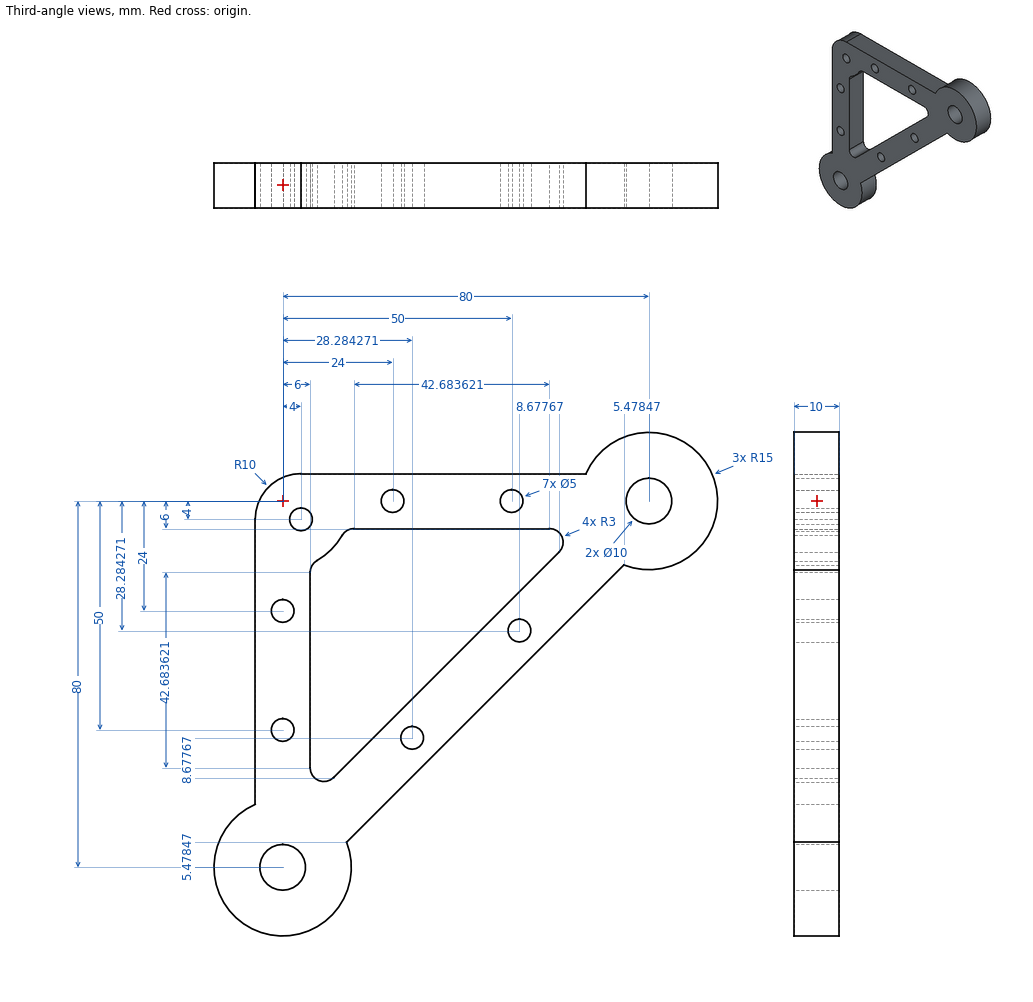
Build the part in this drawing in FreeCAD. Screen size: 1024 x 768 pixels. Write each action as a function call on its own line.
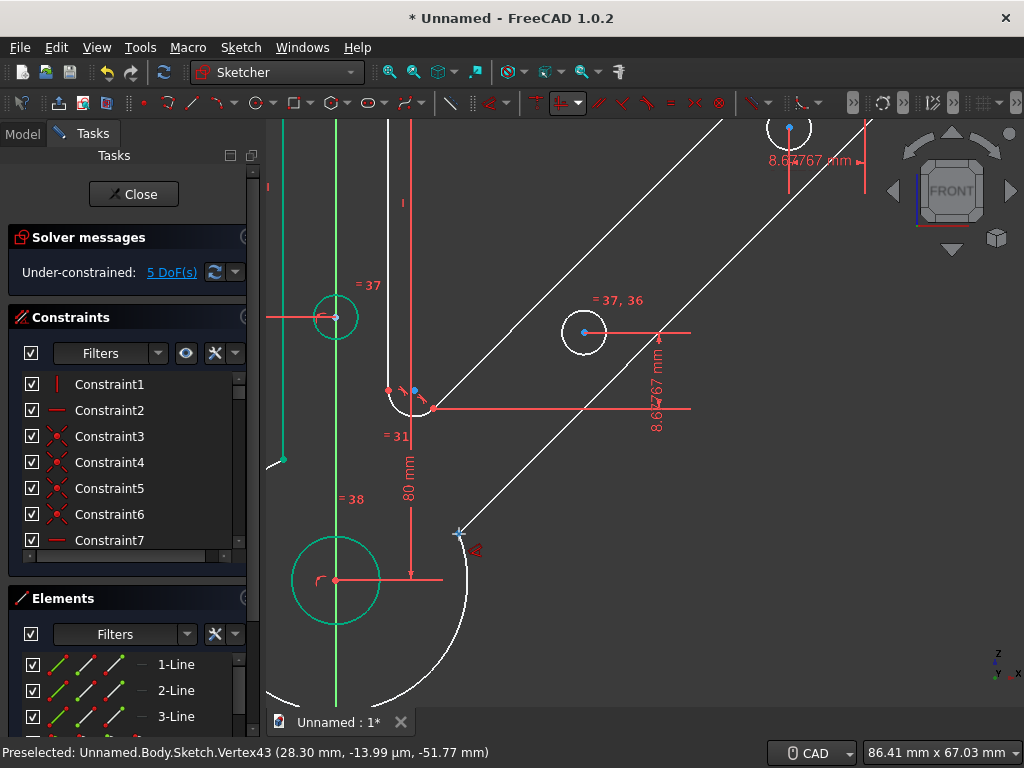
click(459, 534)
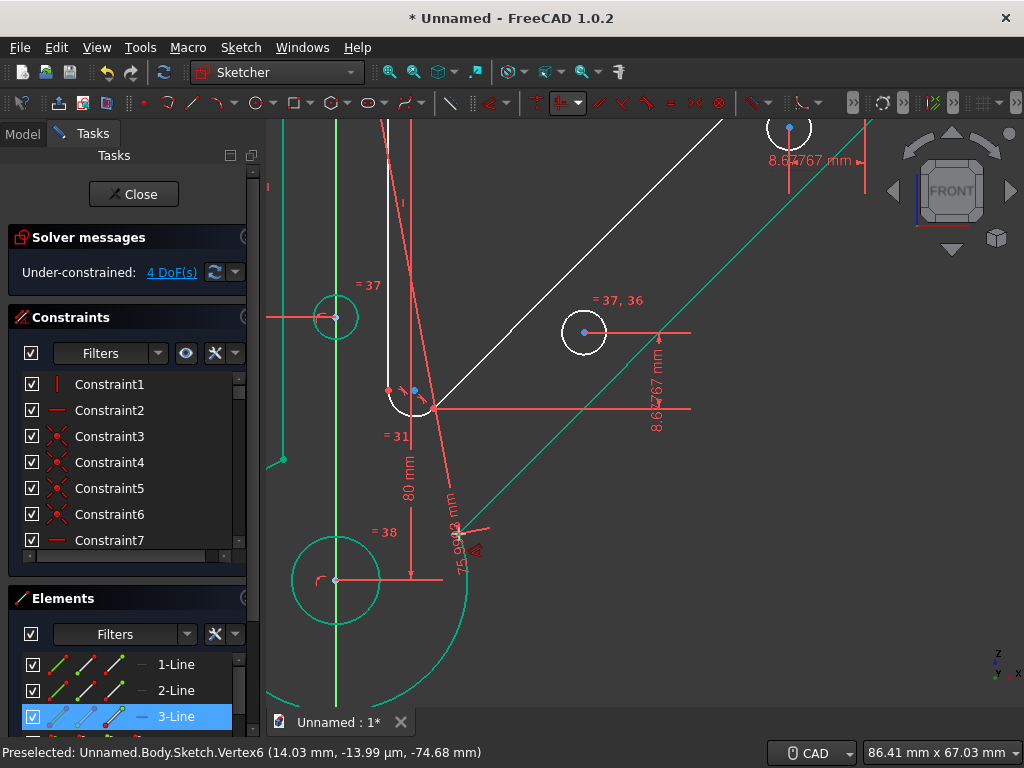
click(336, 580)
click(493, 557)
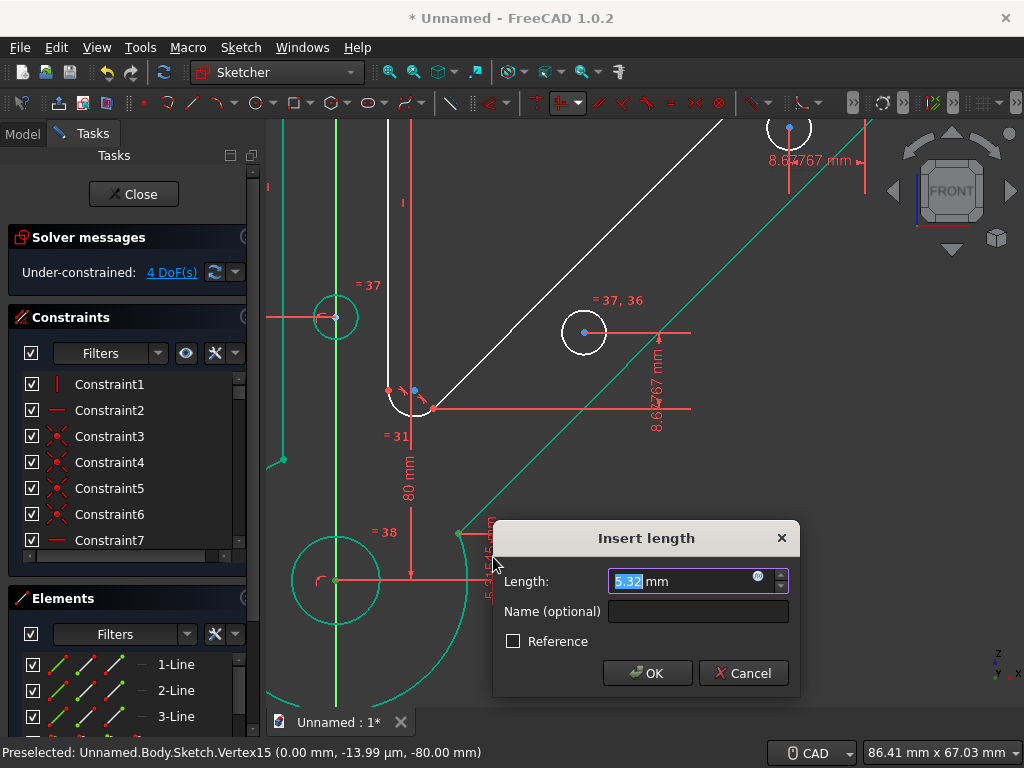
text(5.47847)
key(Return)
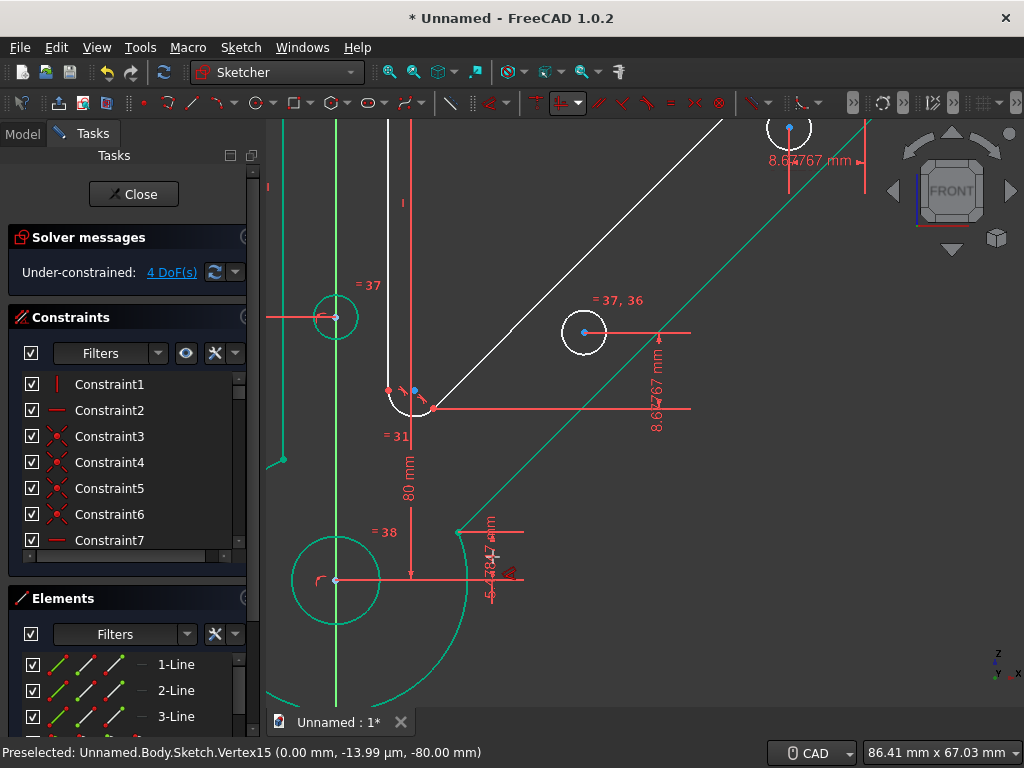
scroll(458, 535, down, 4)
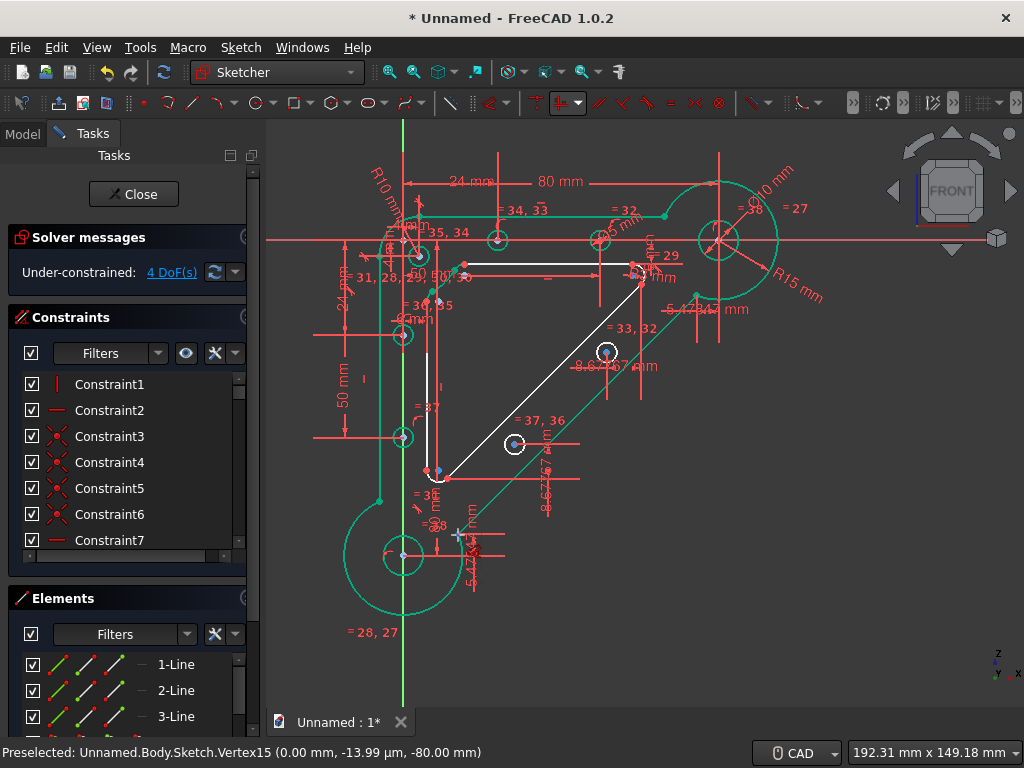
click(582, 264)
click(549, 298)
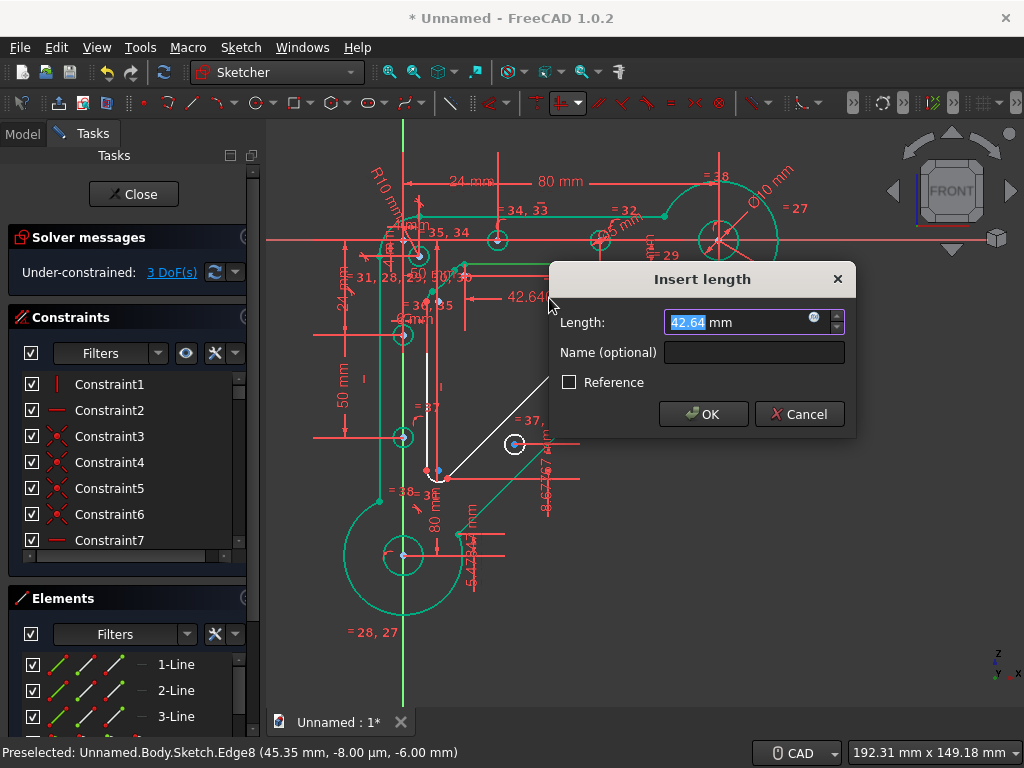
text(42.683621)
key(Return)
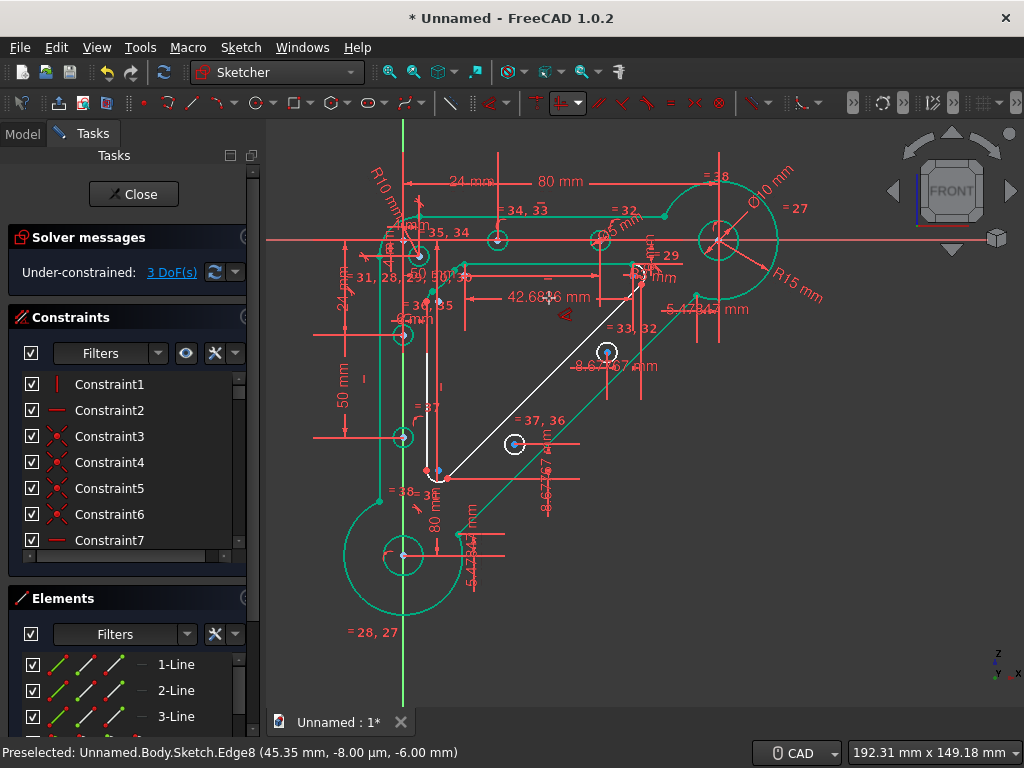
click(427, 352)
click(461, 386)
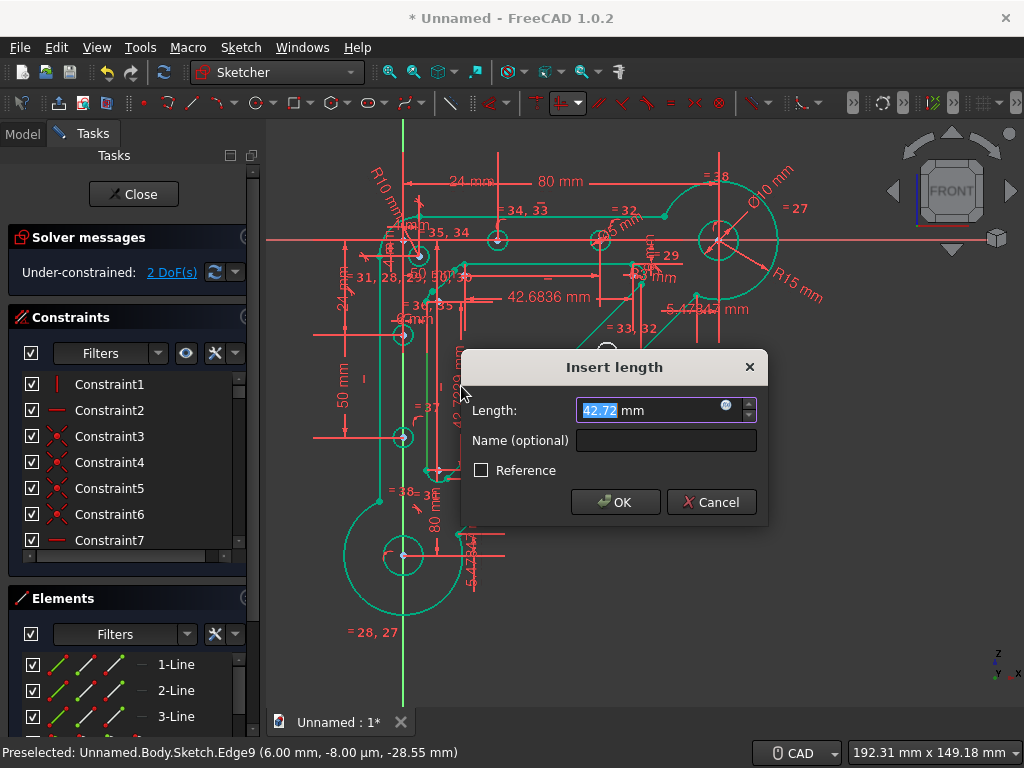
text(42.683621)
key(Return)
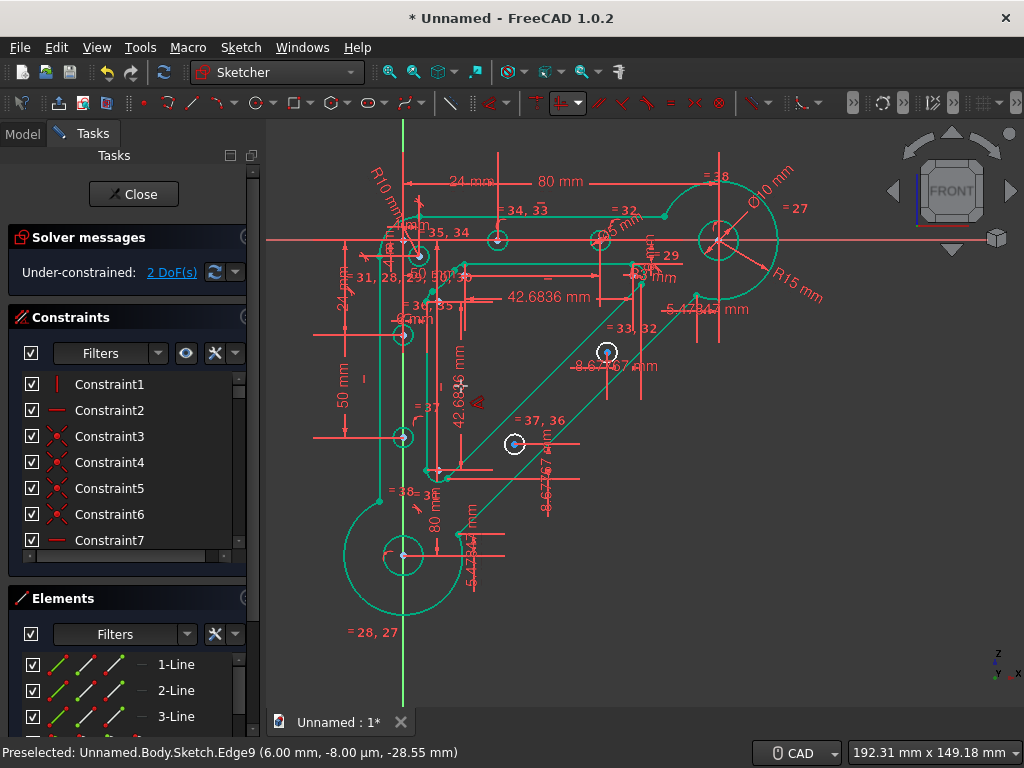
click(607, 352)
click(321, 322)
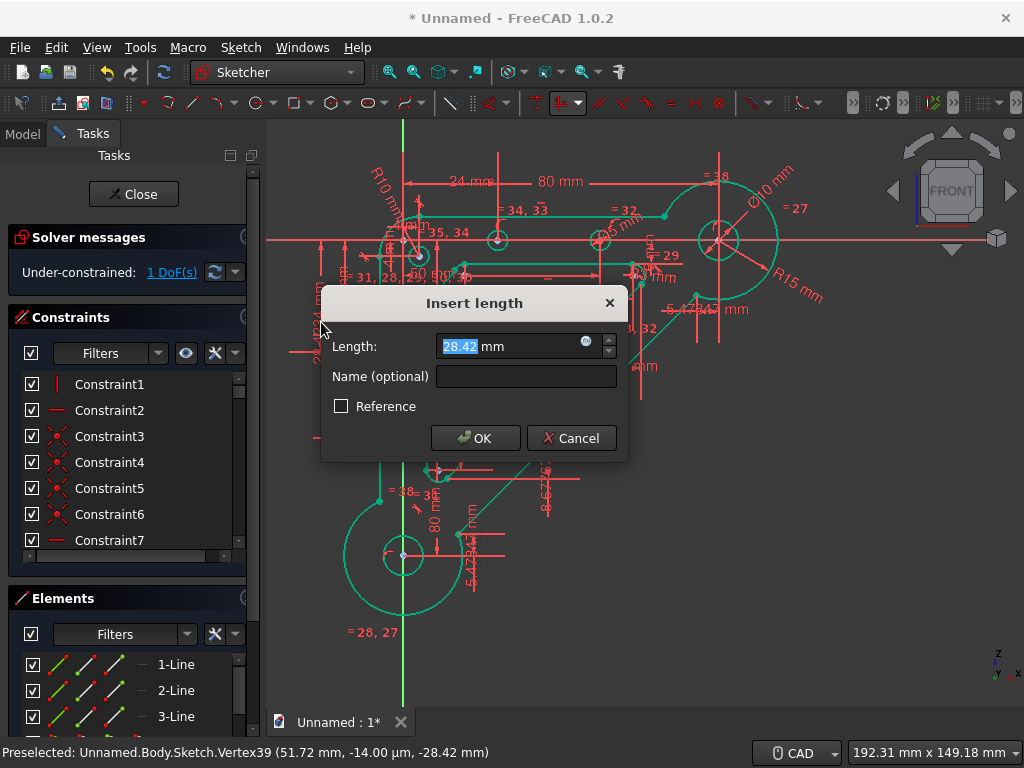
text(28.284271)
key(Return)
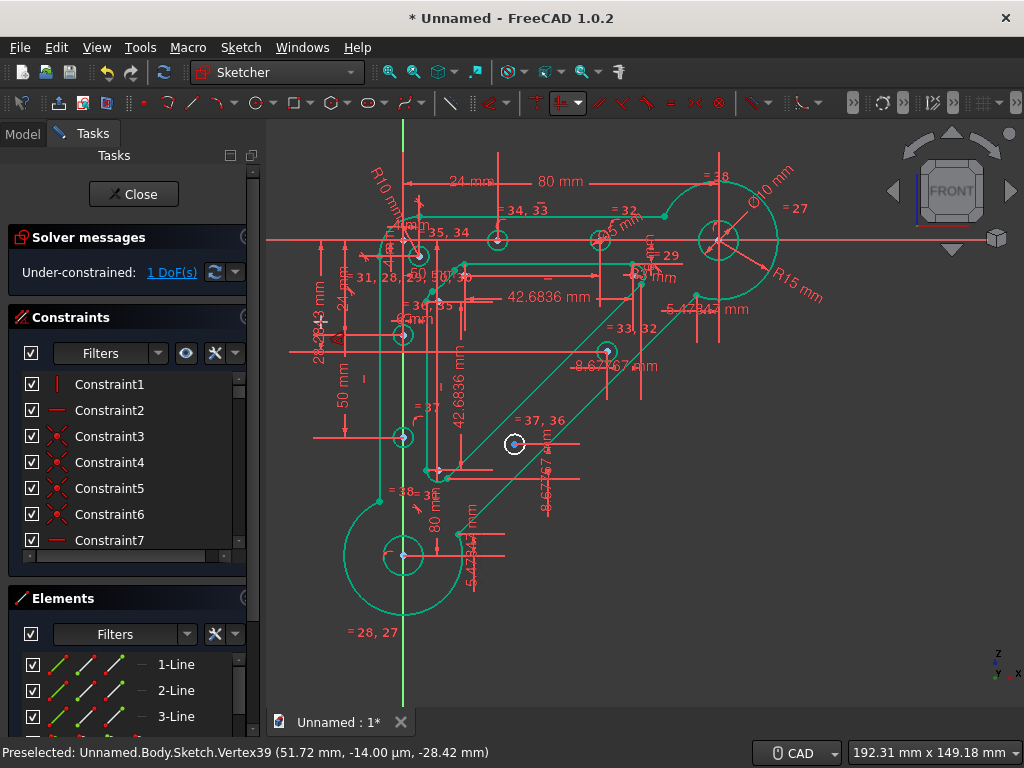
click(515, 444)
click(459, 158)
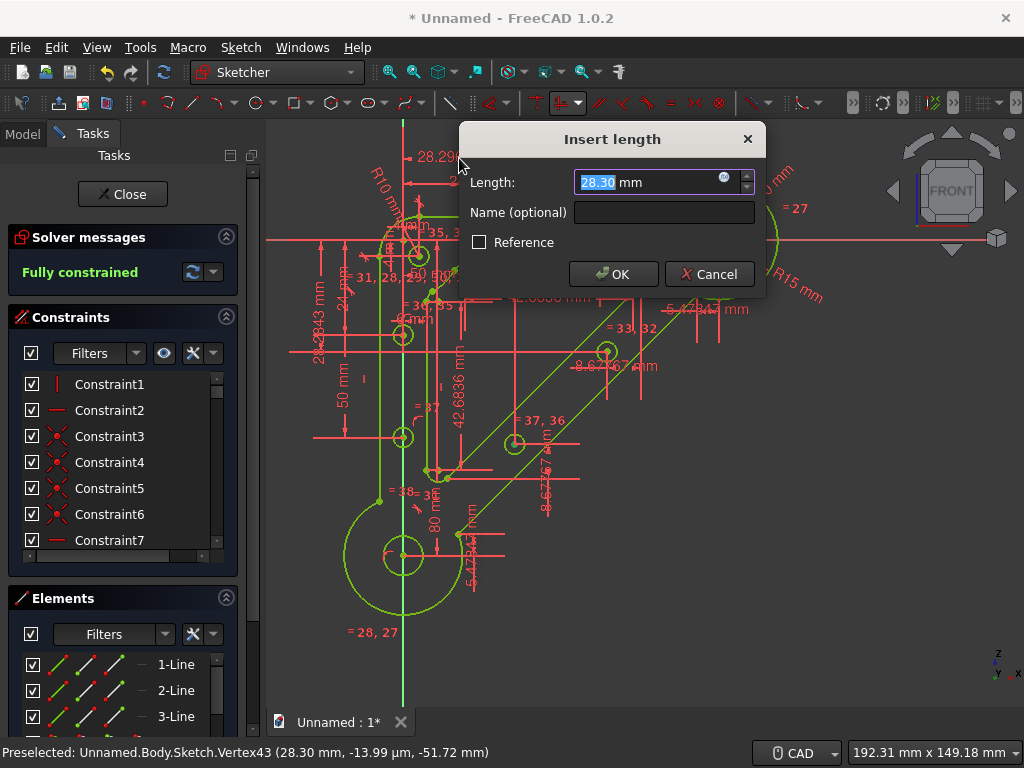
text(28.284271)
key(Return)
key(Escape)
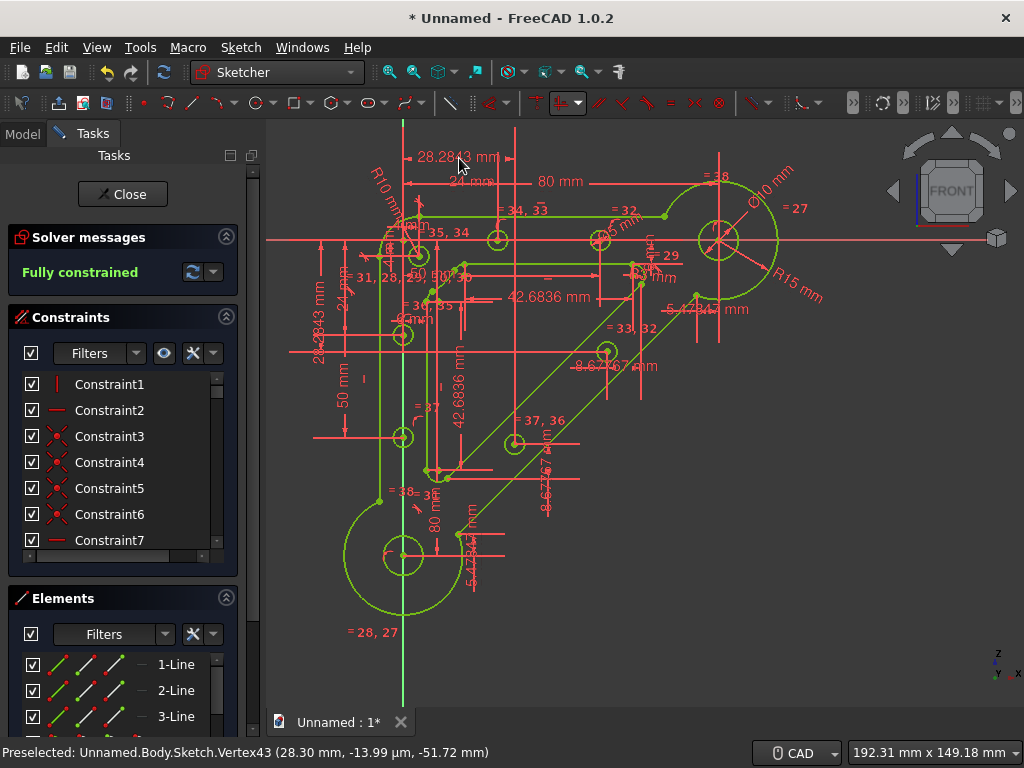
click(123, 194)